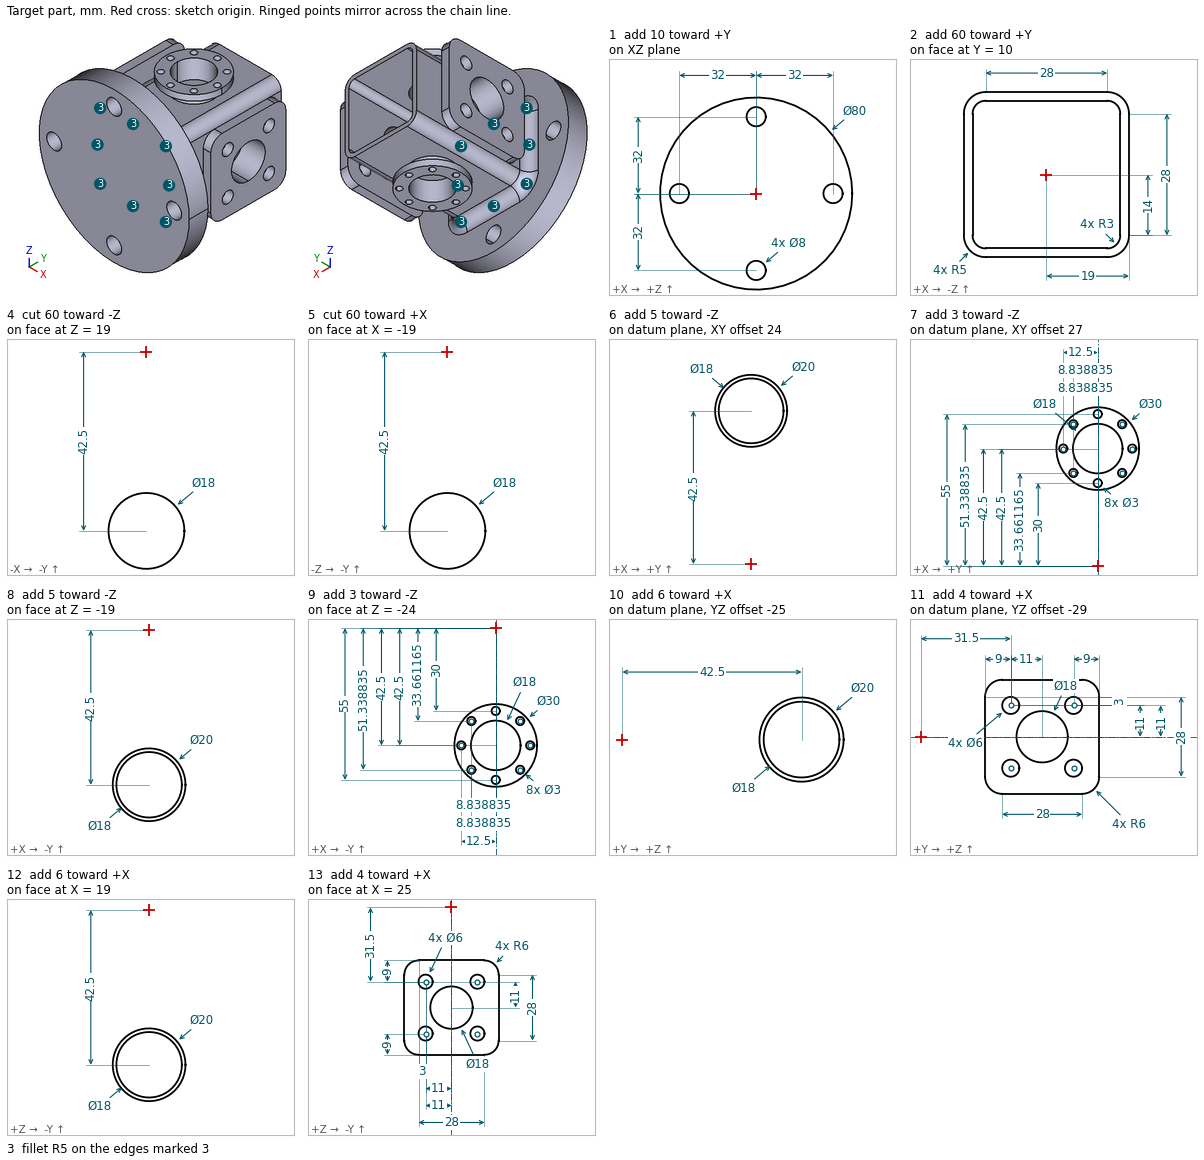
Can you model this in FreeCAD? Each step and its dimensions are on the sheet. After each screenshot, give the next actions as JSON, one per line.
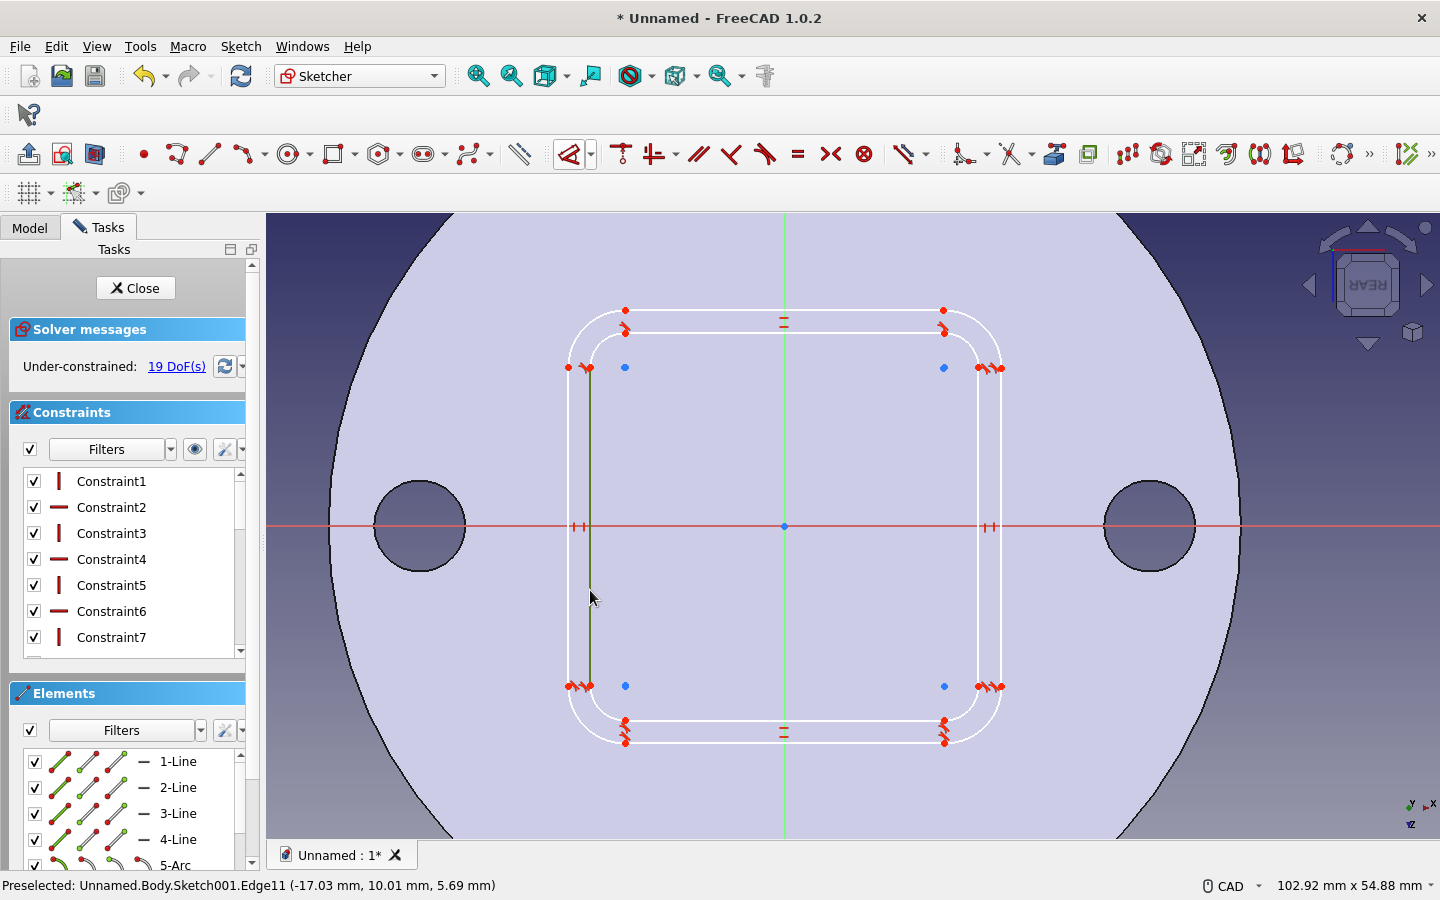
{"action": "left_click", "coordinate": [610, 337]}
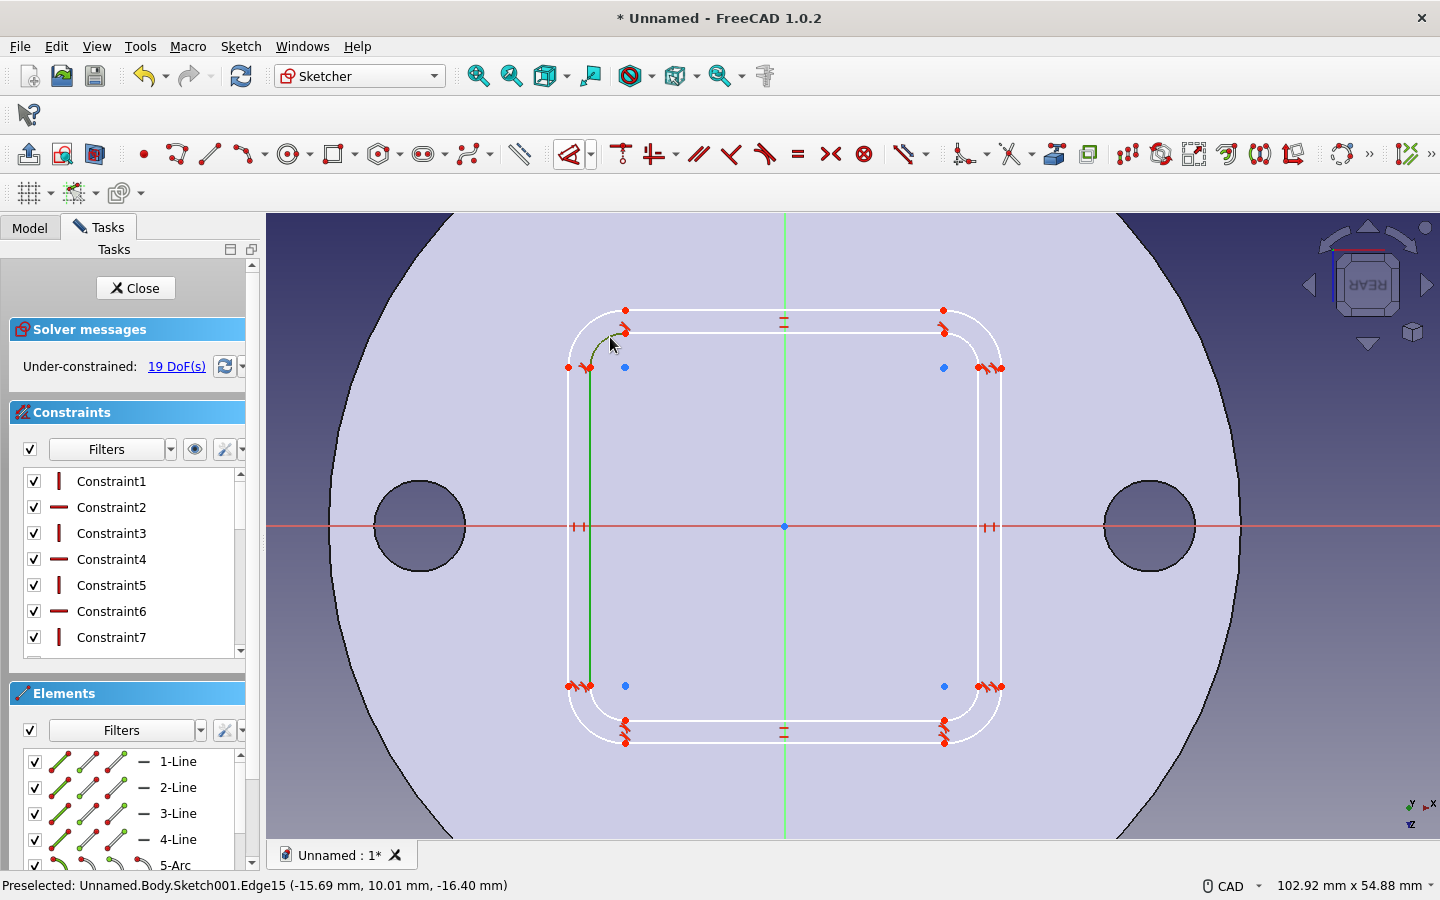
{"action": "key", "text": "t"}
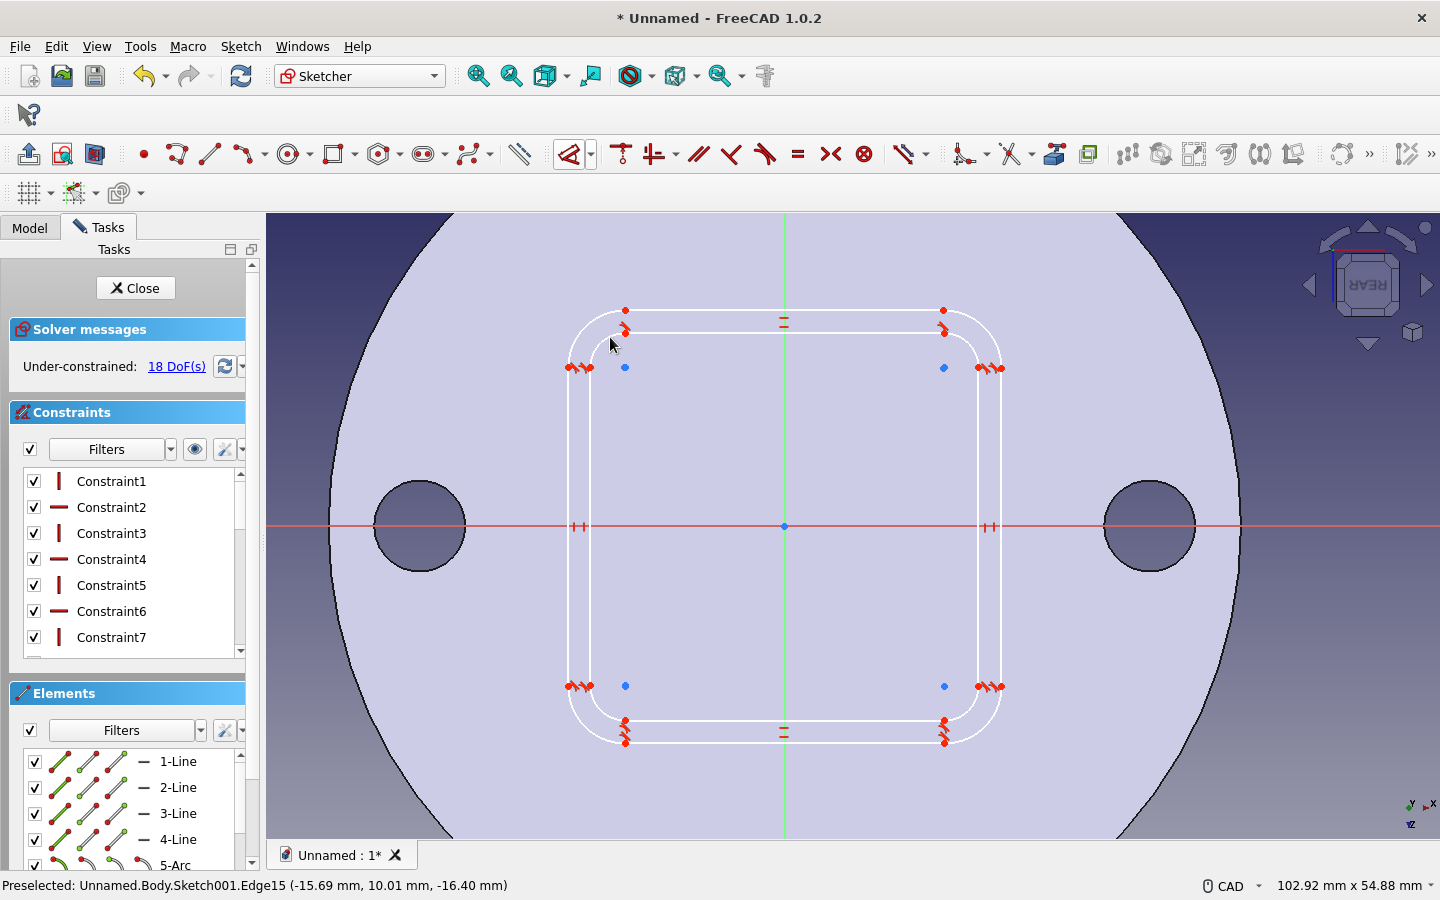
{"action": "left_click", "coordinate": [721, 333]}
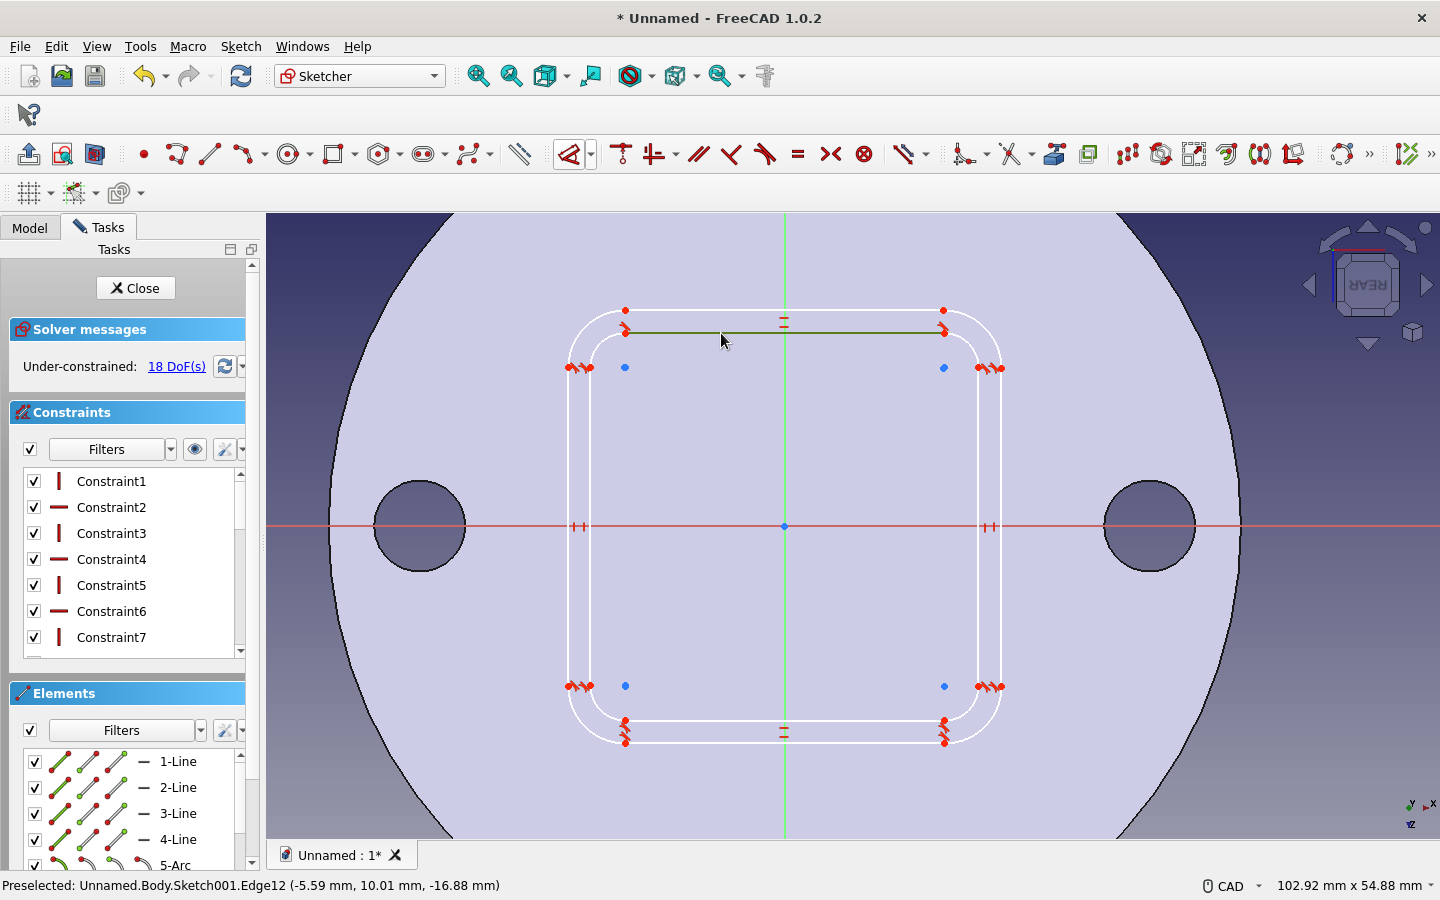
{"action": "left_click", "coordinate": [610, 337]}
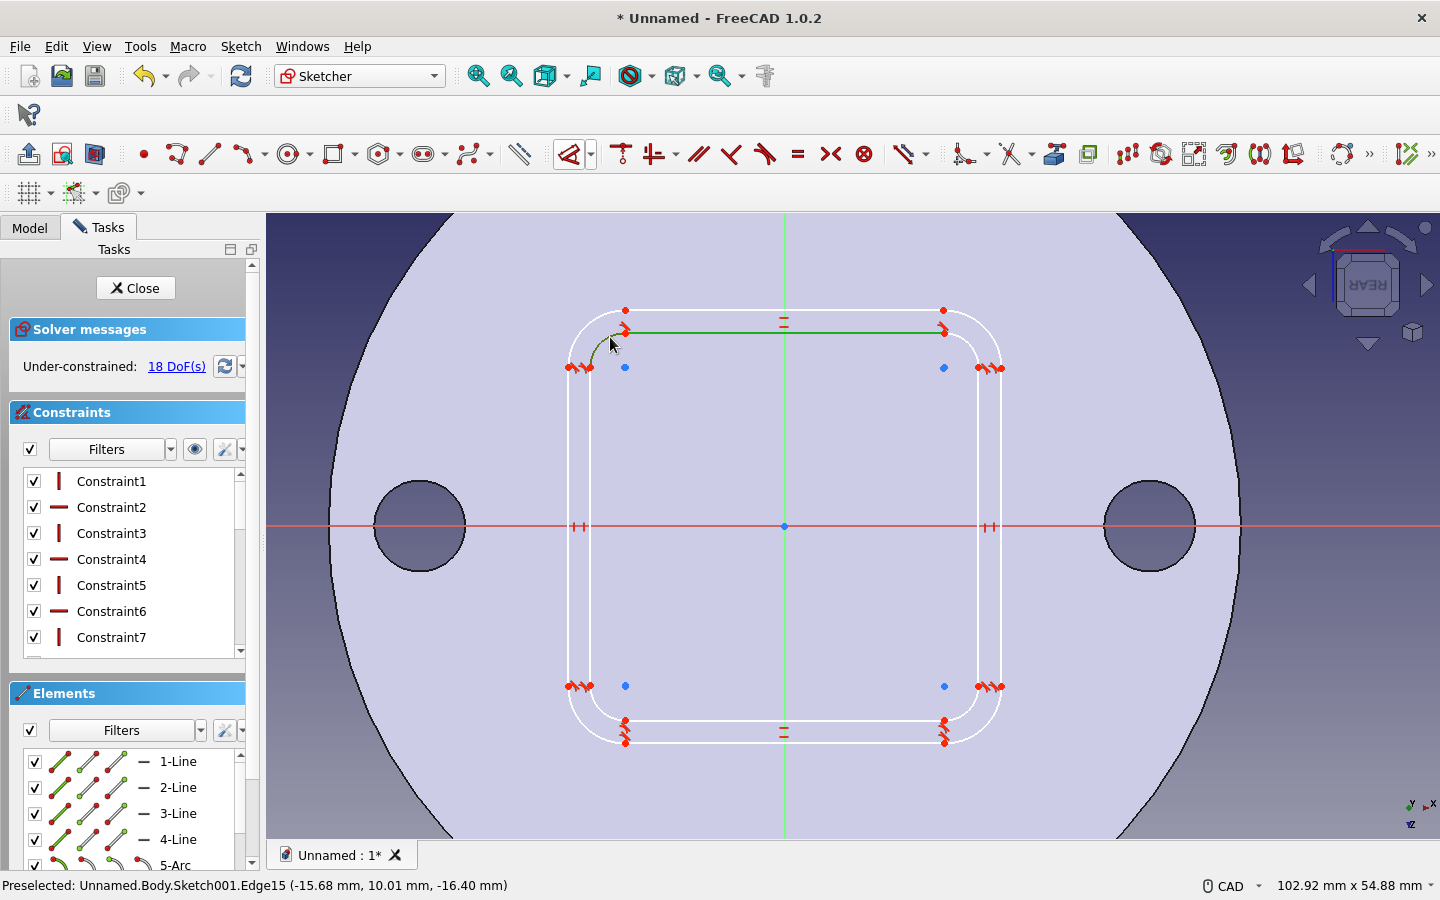
{"action": "key", "text": "t"}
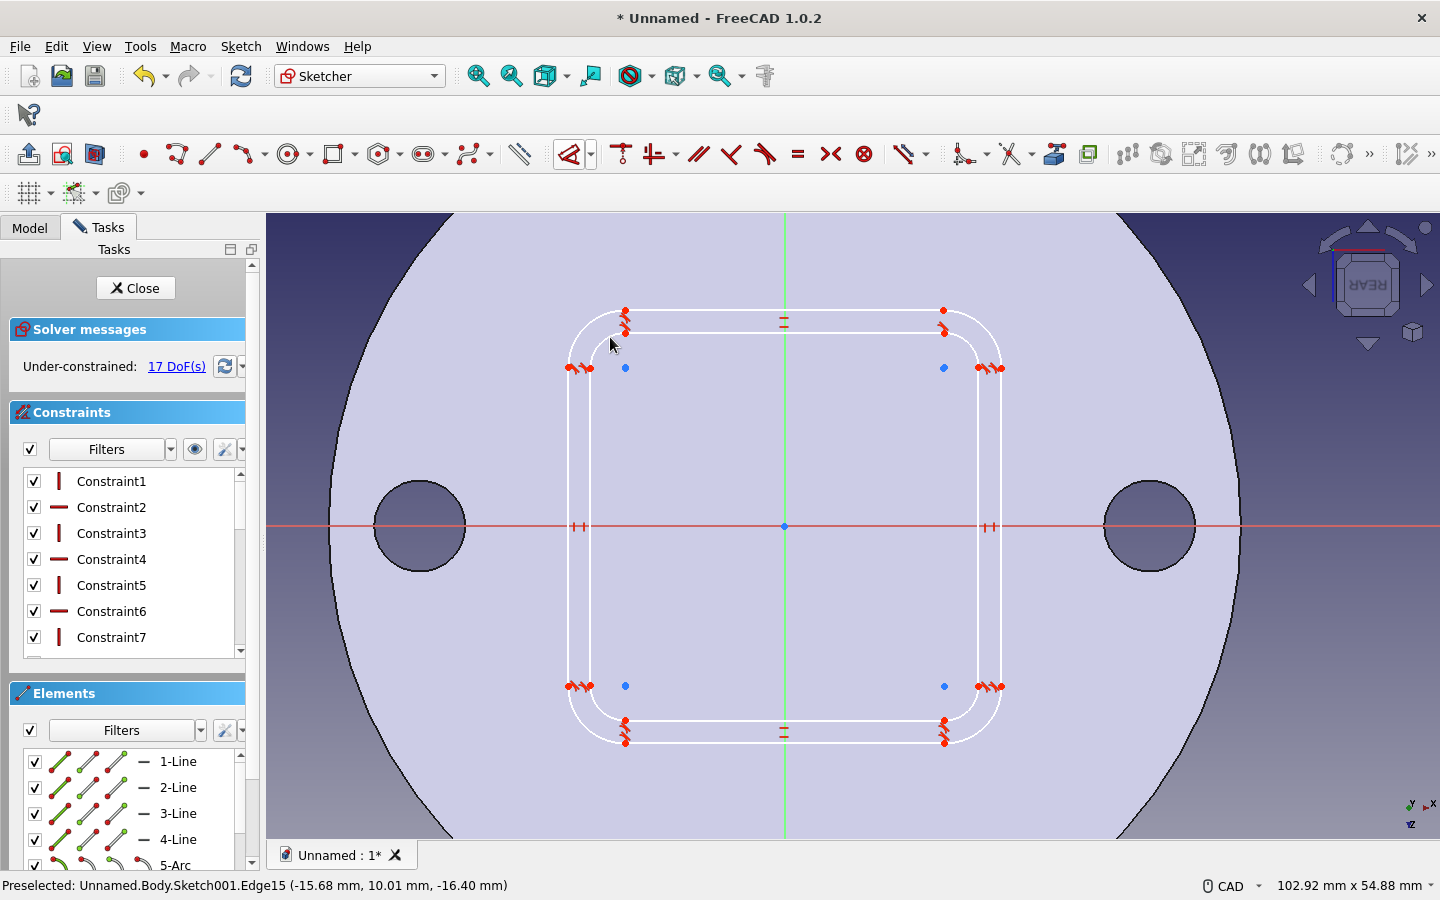
{"action": "left_click", "coordinate": [721, 333]}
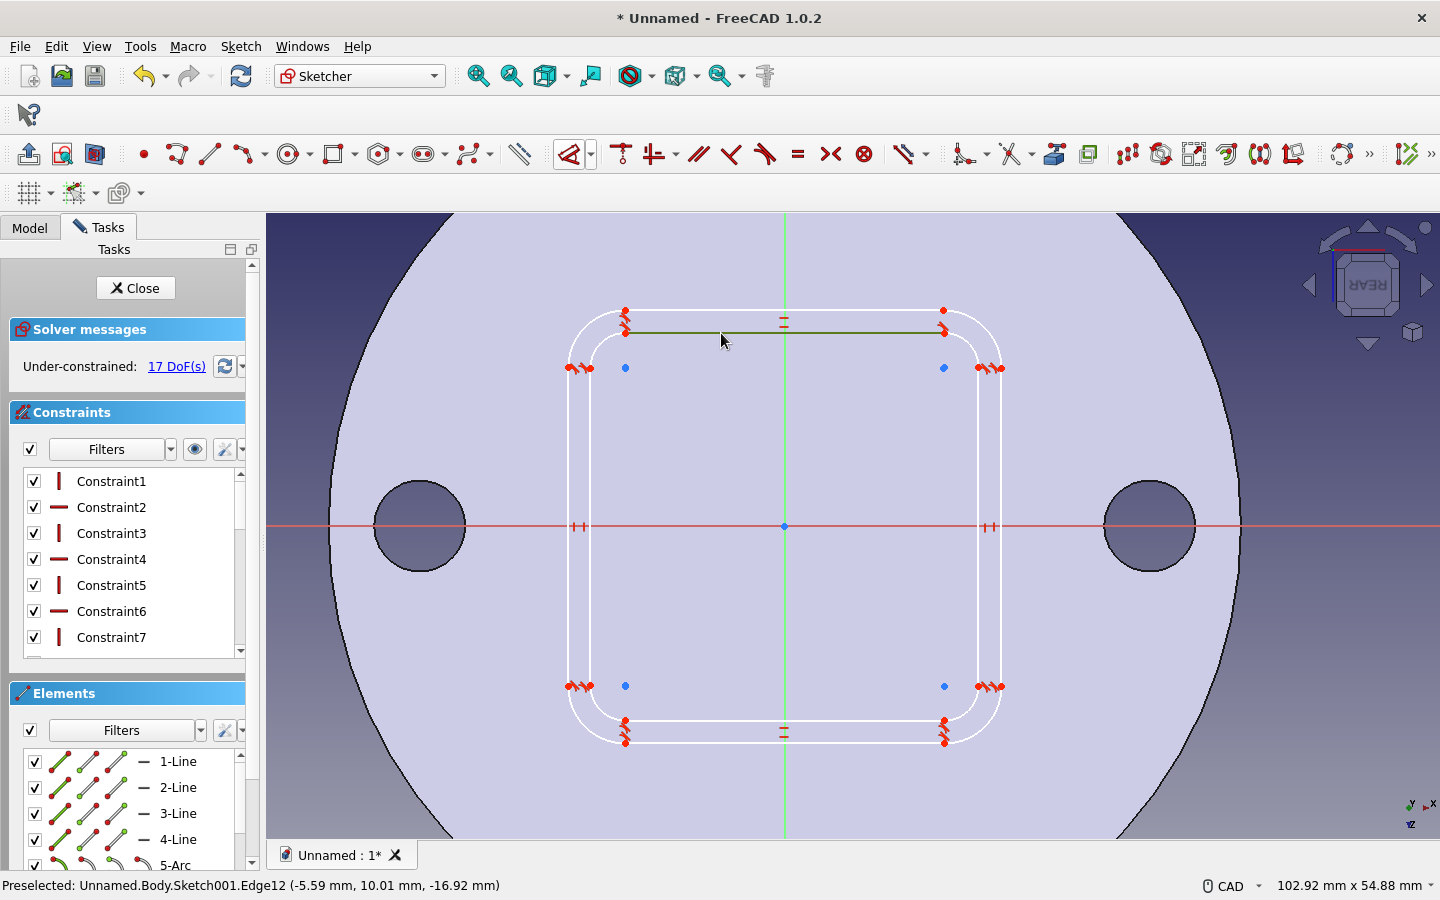
{"action": "left_click", "coordinate": [975, 352]}